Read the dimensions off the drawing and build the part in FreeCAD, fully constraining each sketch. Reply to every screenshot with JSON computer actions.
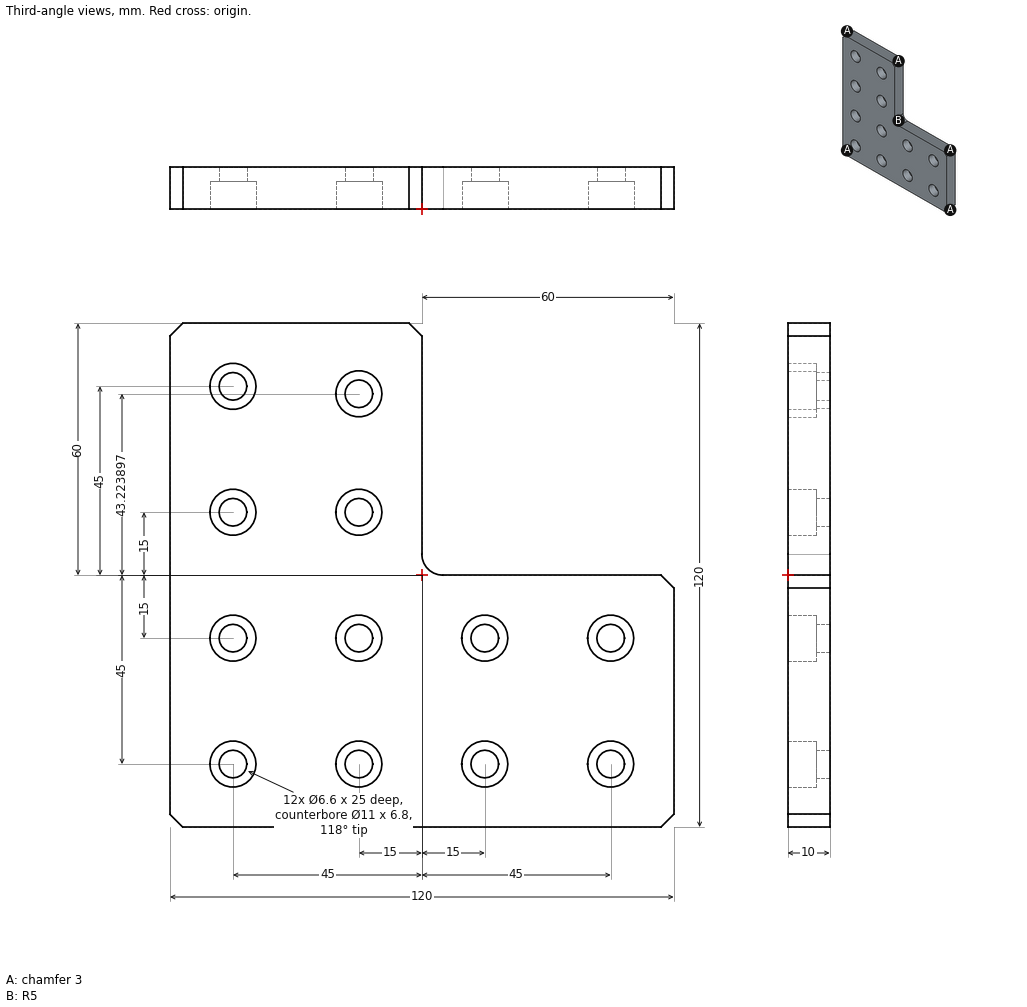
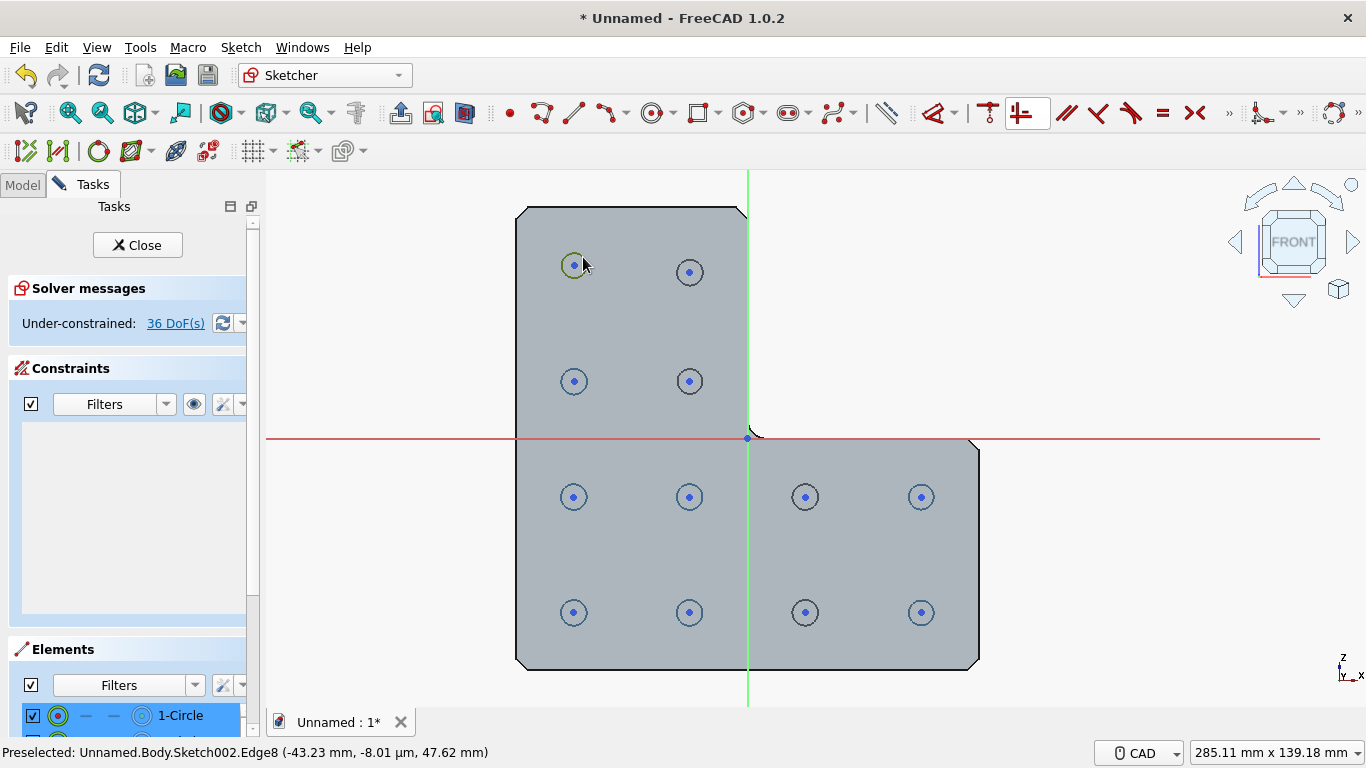
{"action": "left_click", "coordinate": [699, 264]}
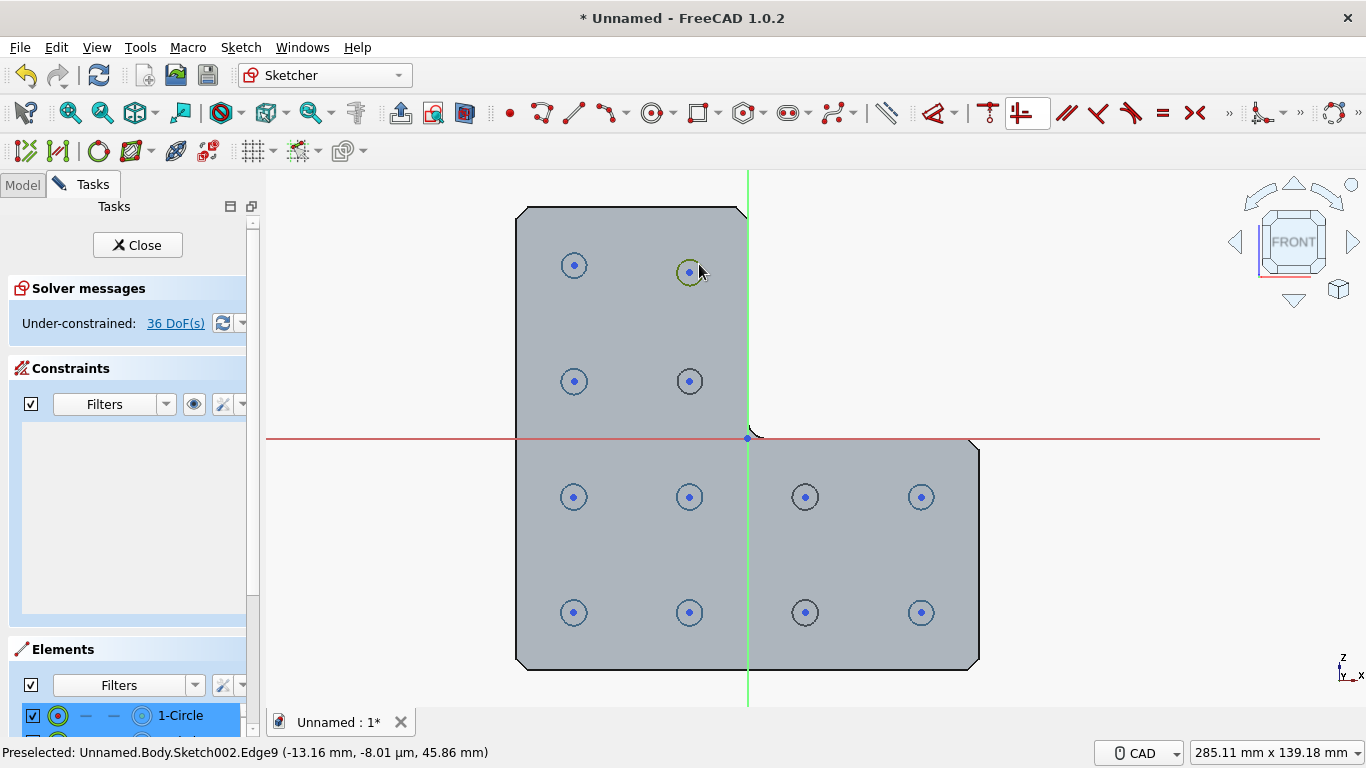
{"action": "left_click", "coordinate": [699, 373]}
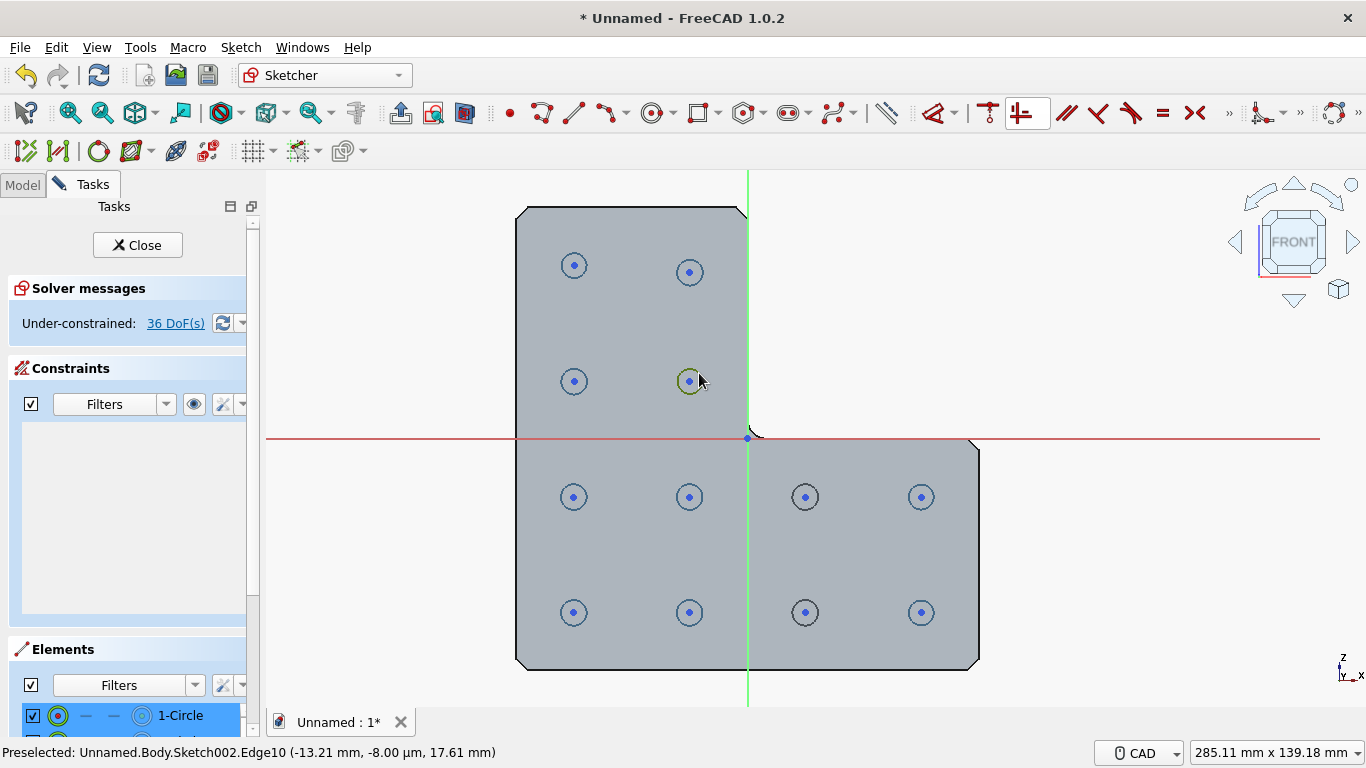
{"action": "left_click", "coordinate": [814, 604]}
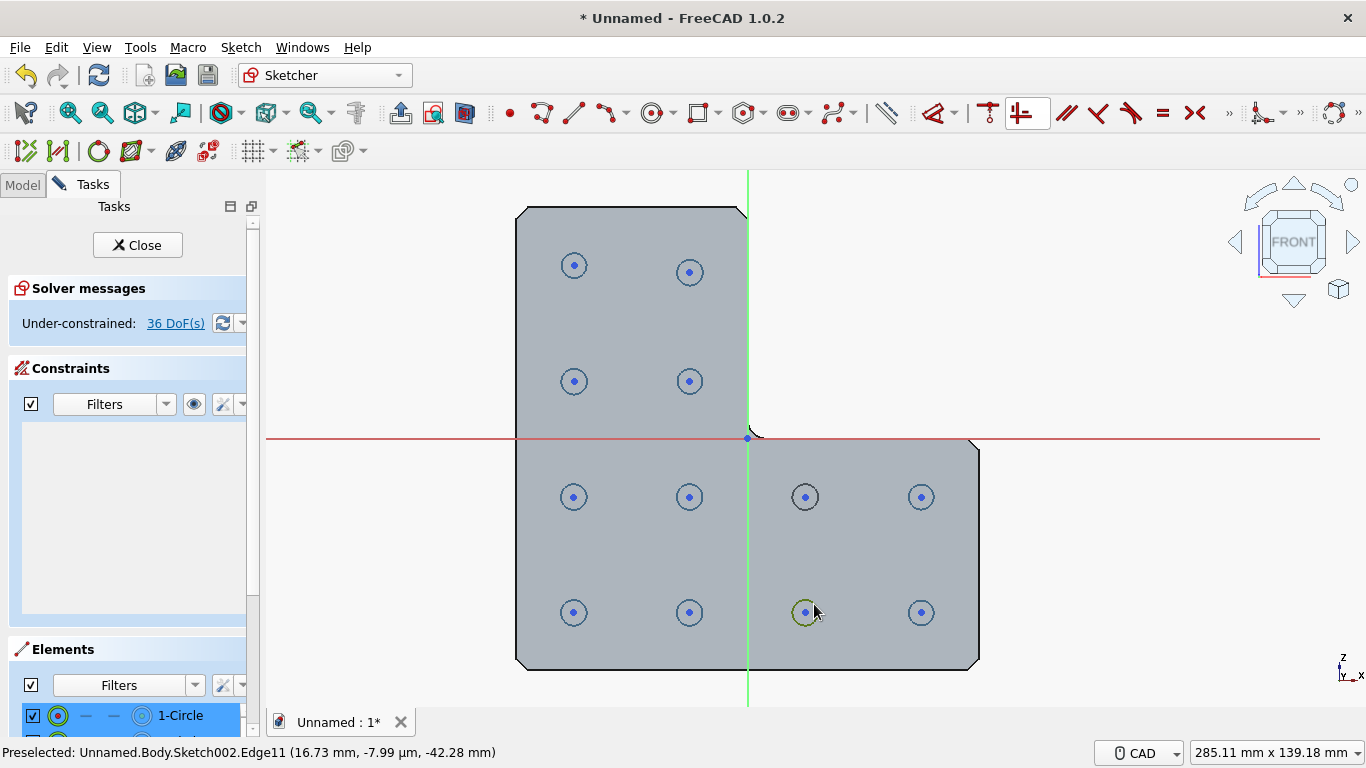
{"action": "left_click", "coordinate": [814, 488]}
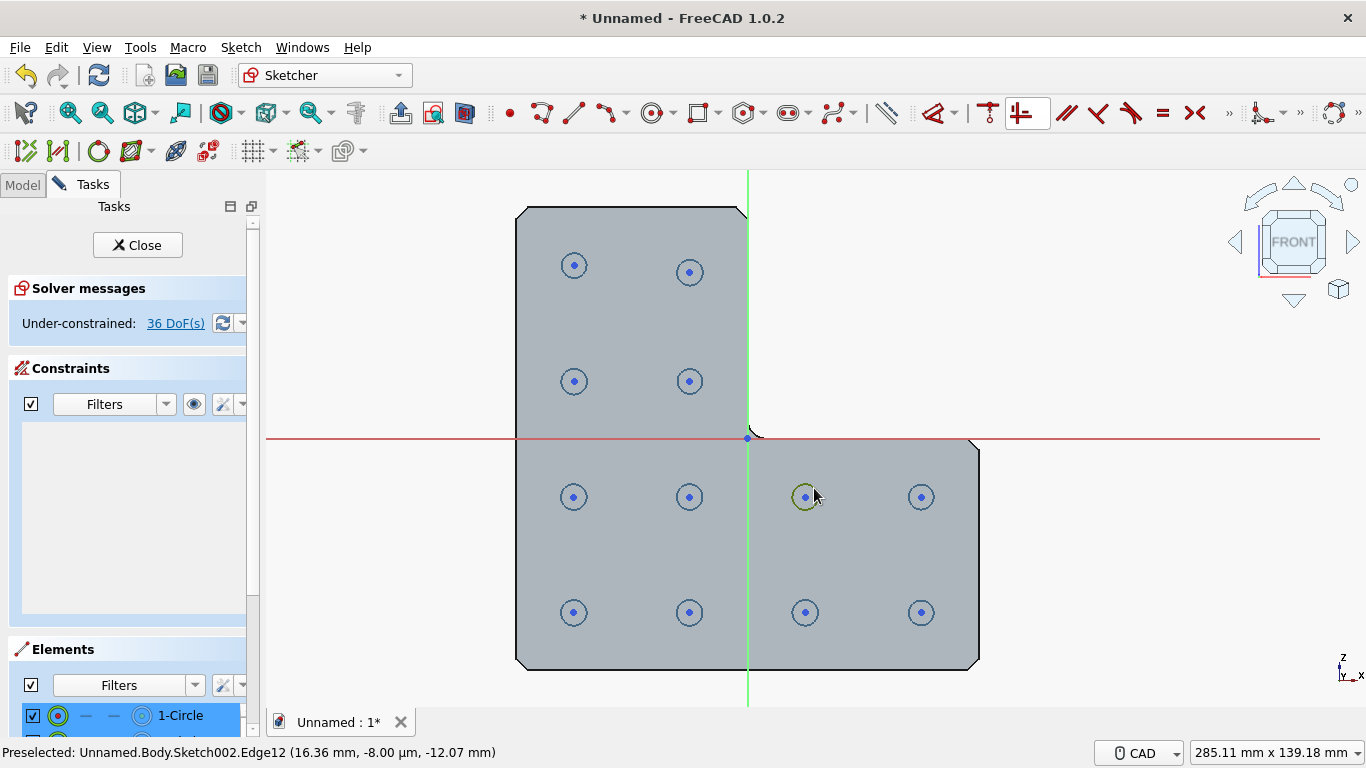
{"action": "left_click", "coordinate": [1164, 114]}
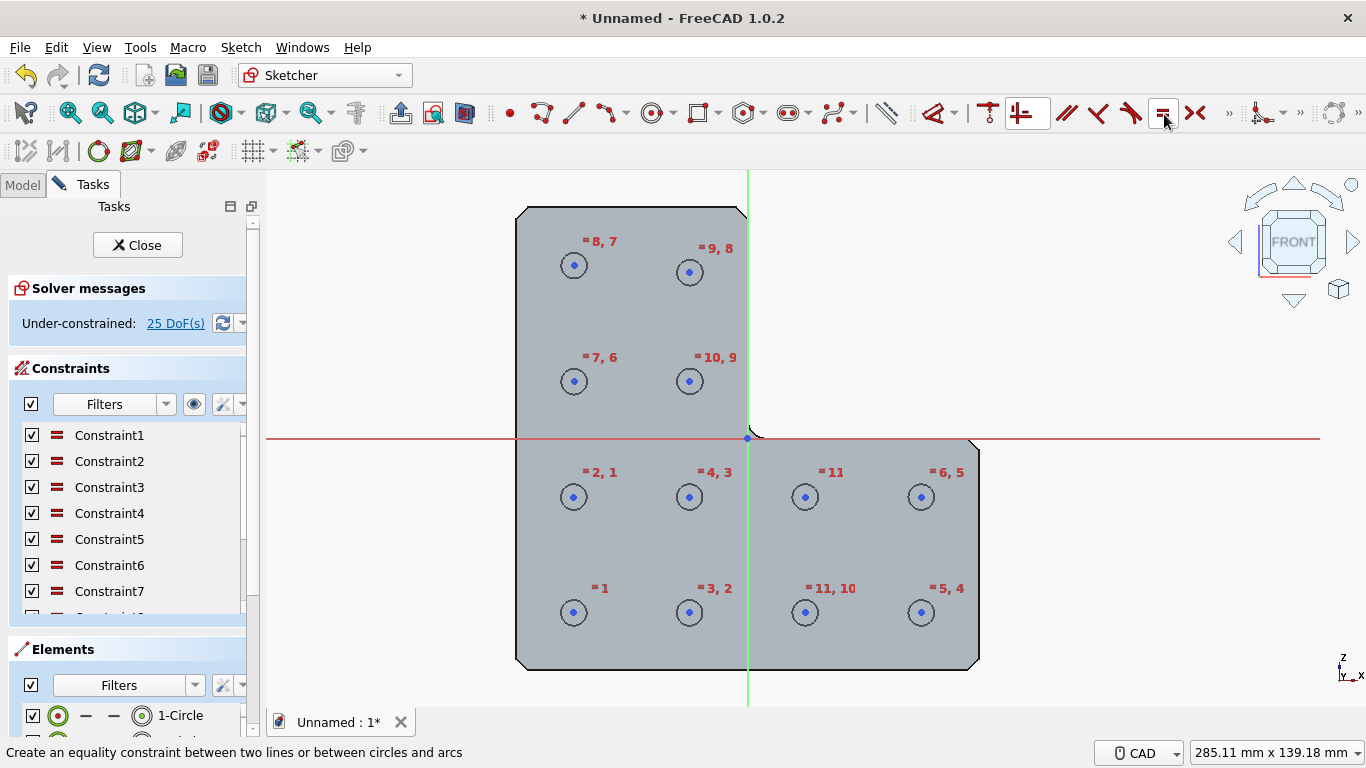
{"action": "left_click", "coordinate": [934, 114]}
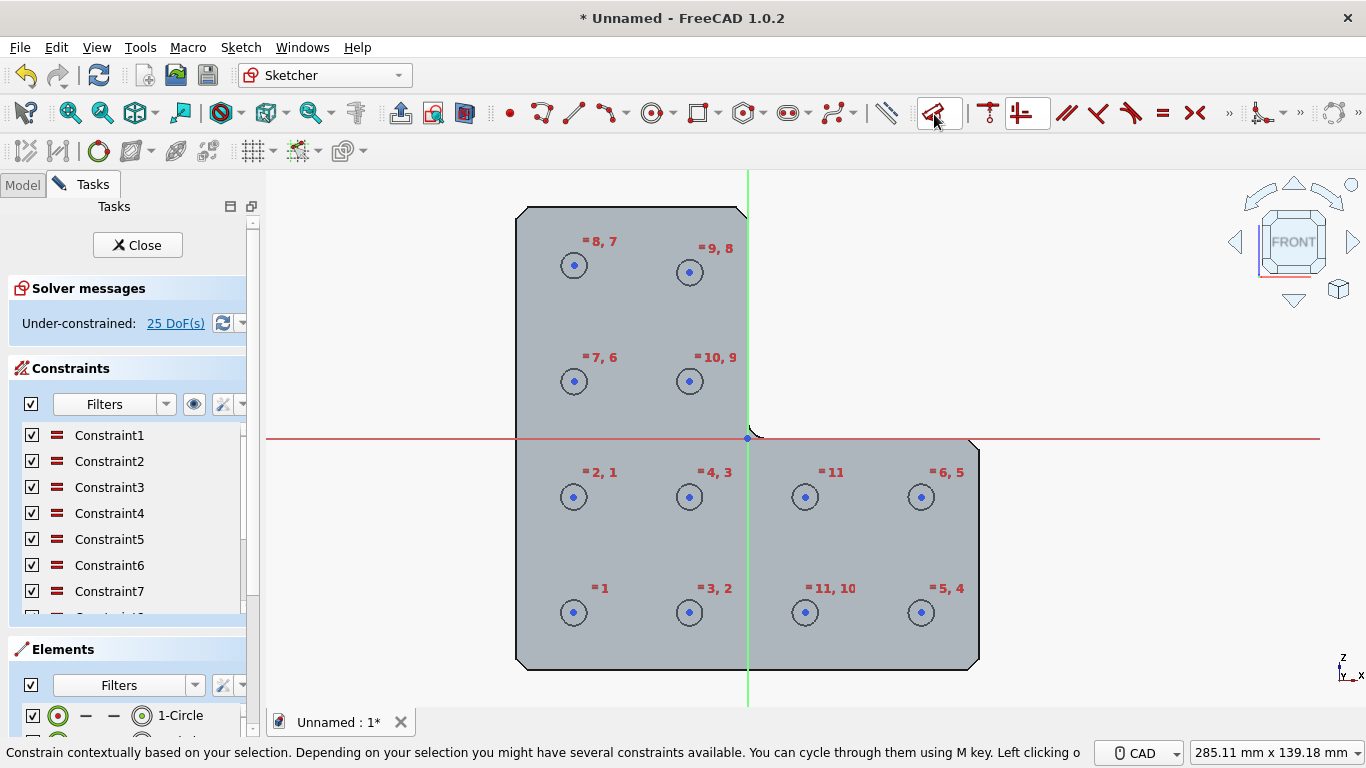
{"action": "scroll", "coordinate": [583, 604], "scroll_direction": "up", "scroll_amount": 3}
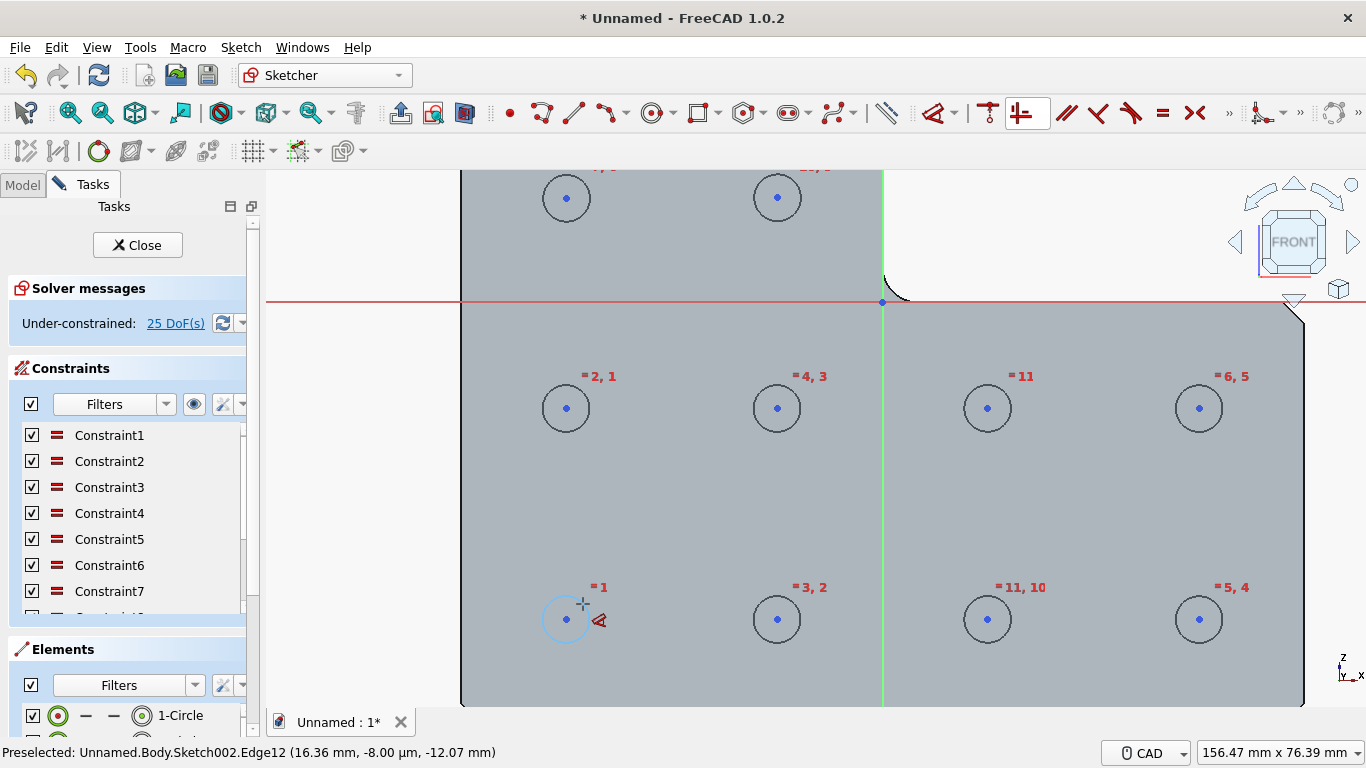
{"action": "left_click", "coordinate": [582, 603]}
{"action": "left_click", "coordinate": [604, 580]}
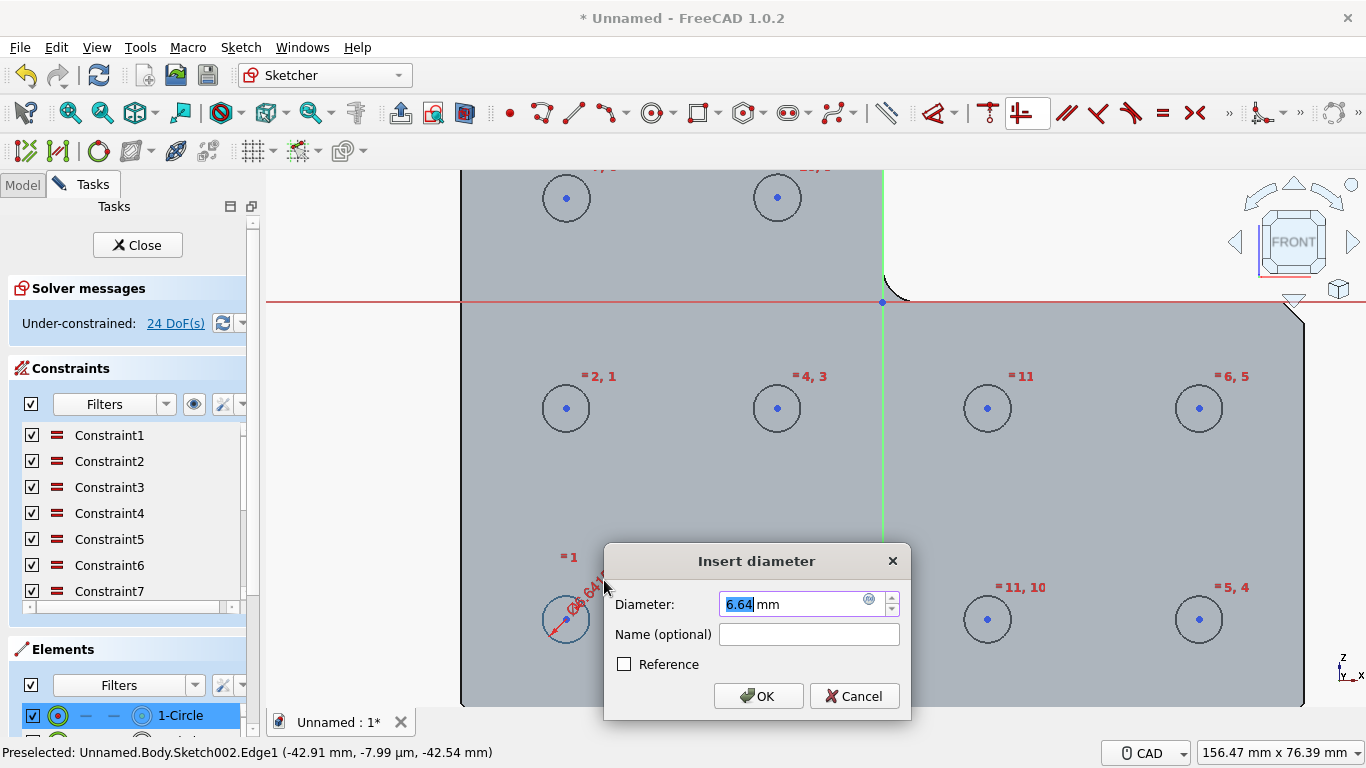
{"action": "type", "text": "6.6"}
{"action": "key", "text": "Return"}